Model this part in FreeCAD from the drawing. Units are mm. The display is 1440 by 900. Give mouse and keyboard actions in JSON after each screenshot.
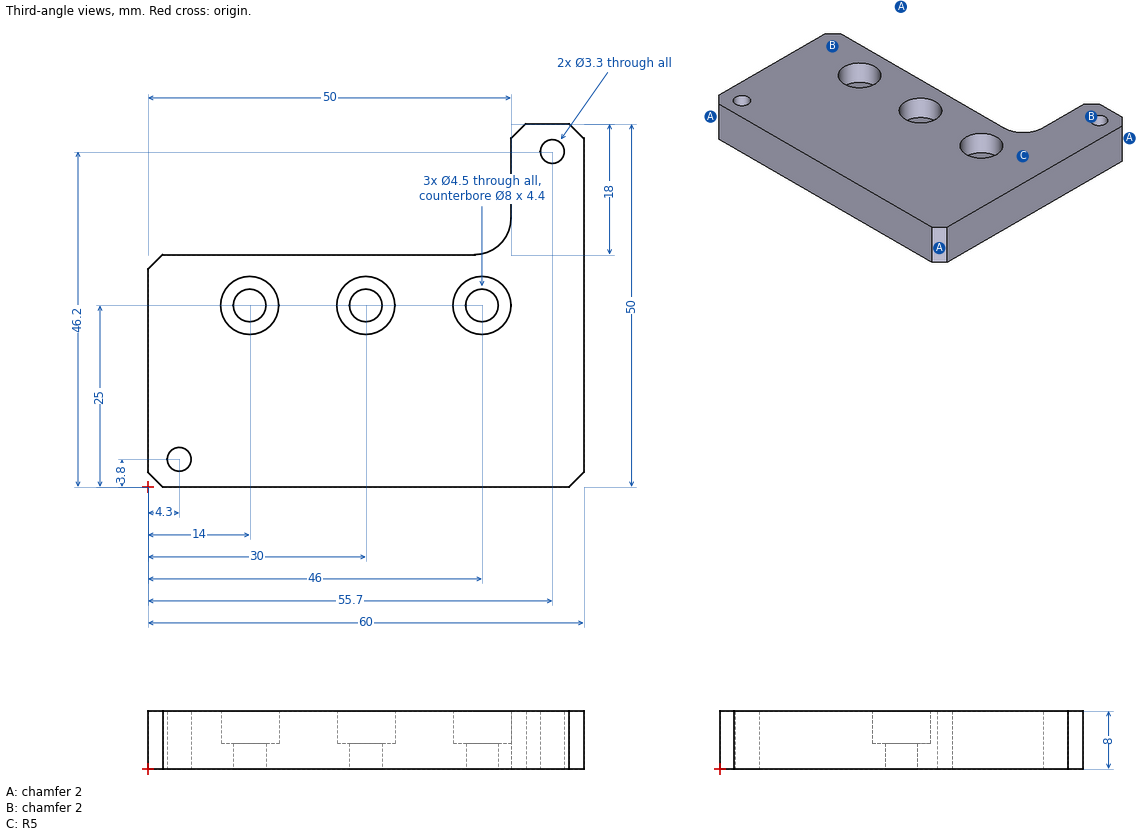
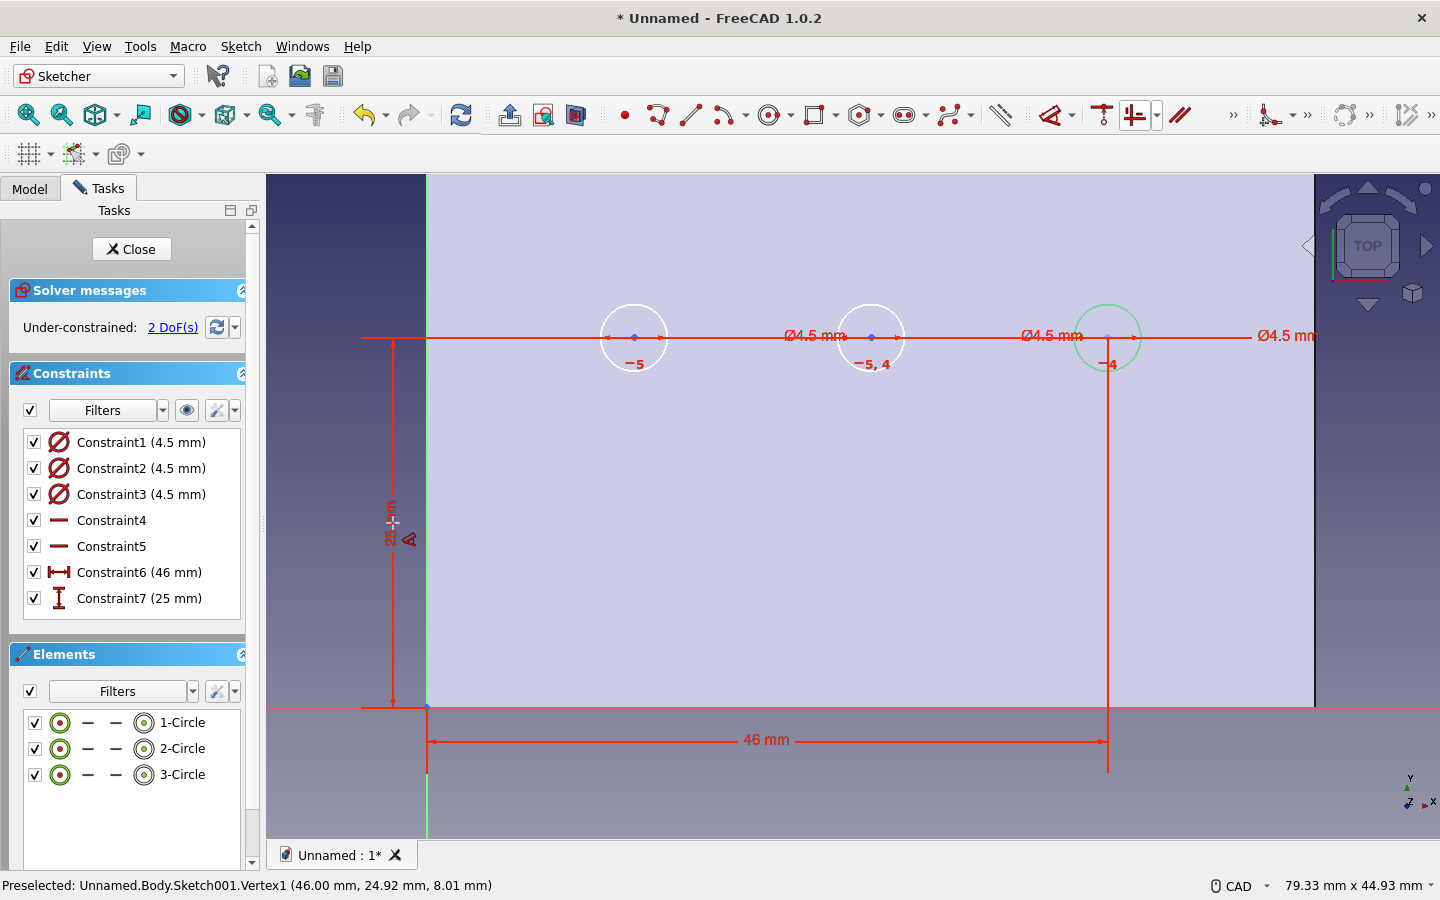
{"action": "left_click", "coordinate": [871, 338]}
{"action": "left_click", "coordinate": [649, 742]}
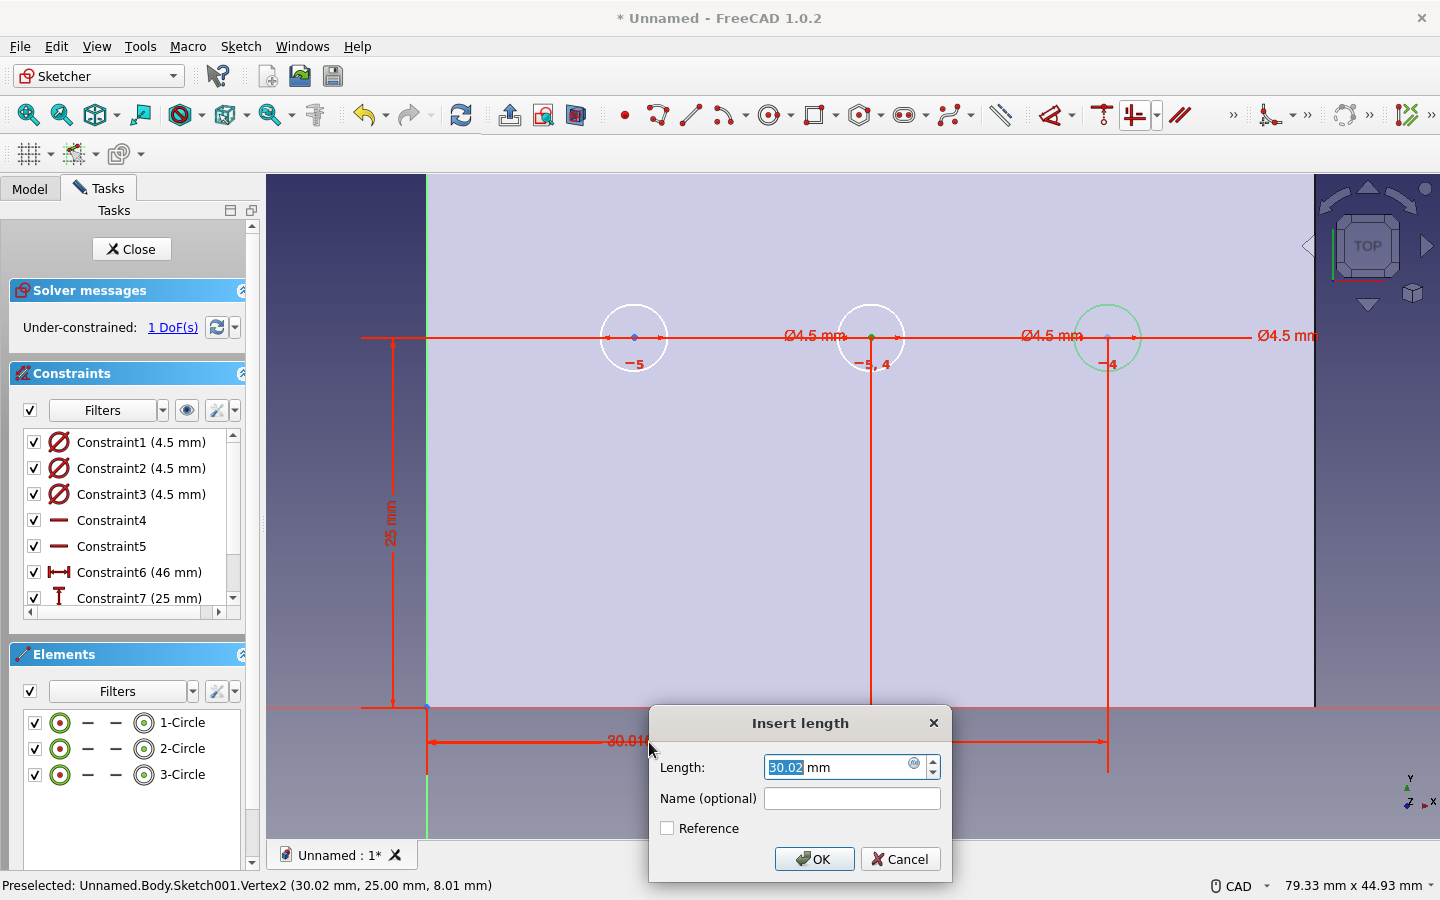
{"action": "type", "text": "30"}
{"action": "key", "text": "Return"}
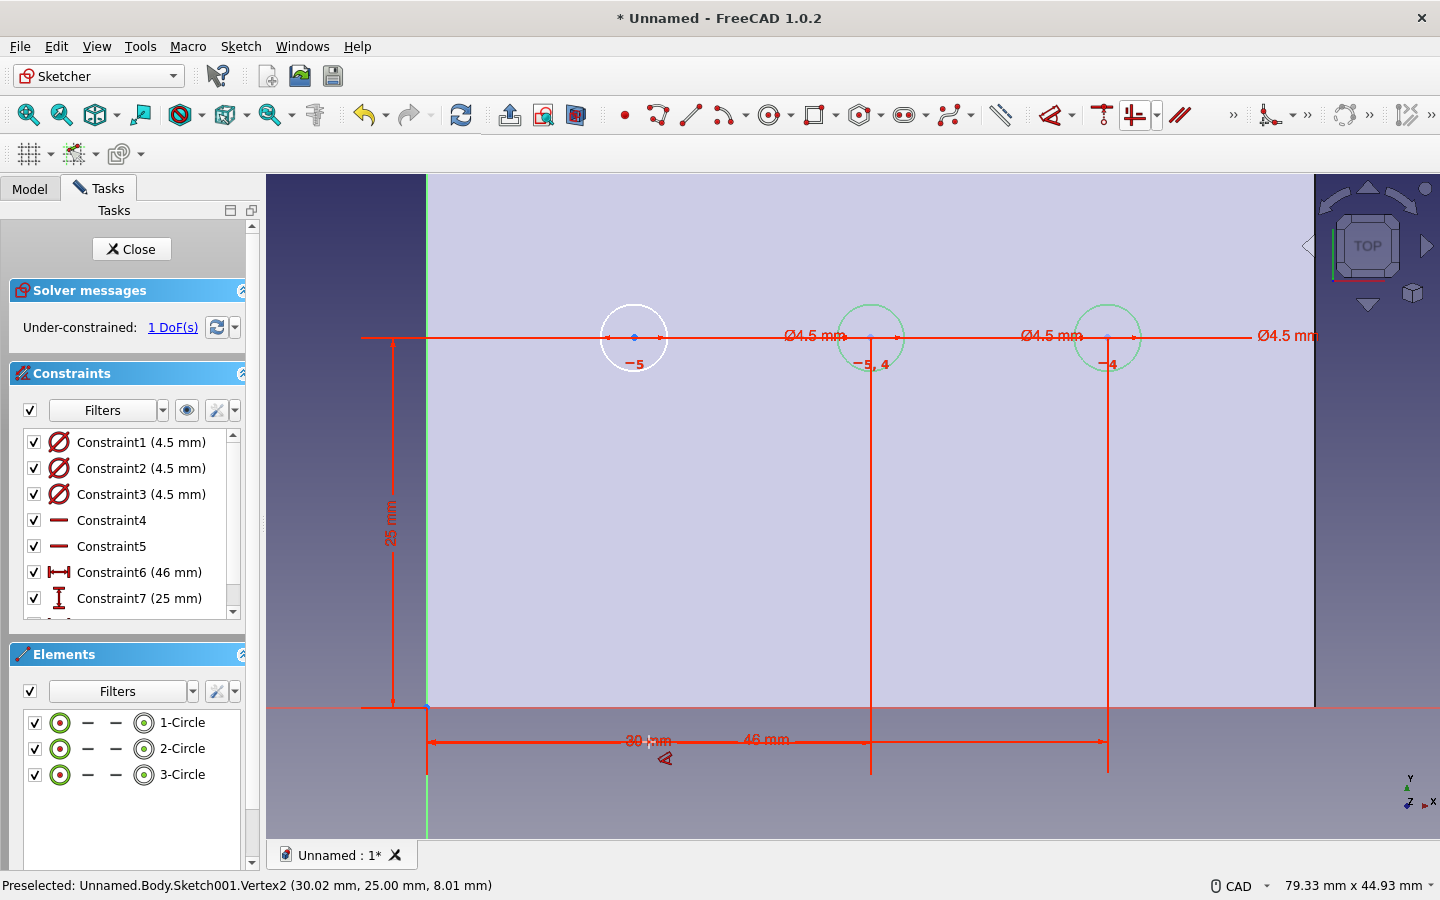
{"action": "left_click", "coordinate": [634, 338]}
{"action": "left_click", "coordinate": [530, 742]}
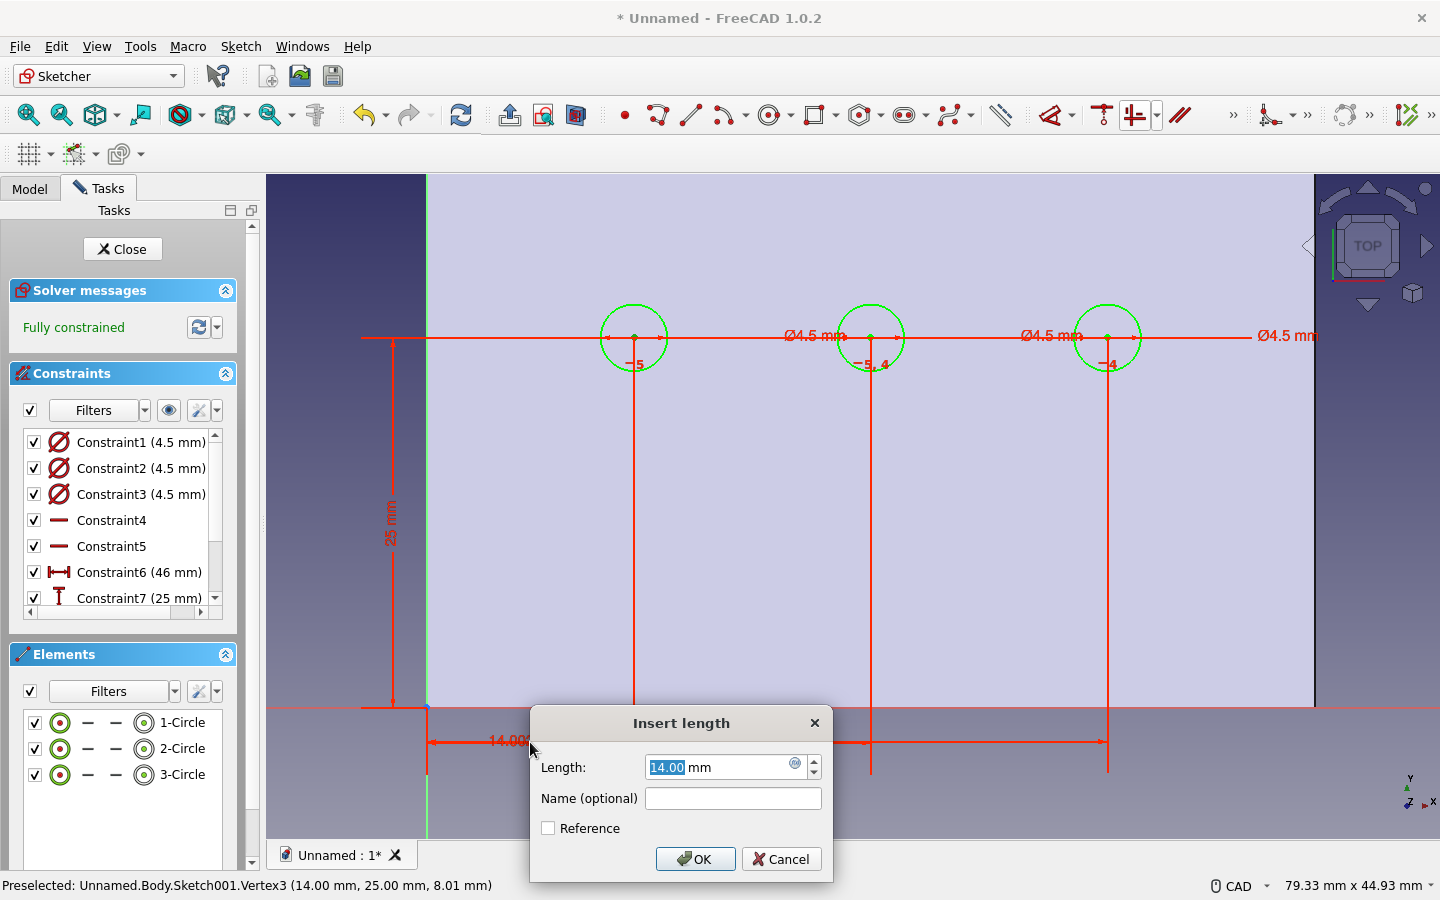
{"action": "type", "text": "14"}
{"action": "key", "text": "Return"}
{"action": "key", "text": "Escape"}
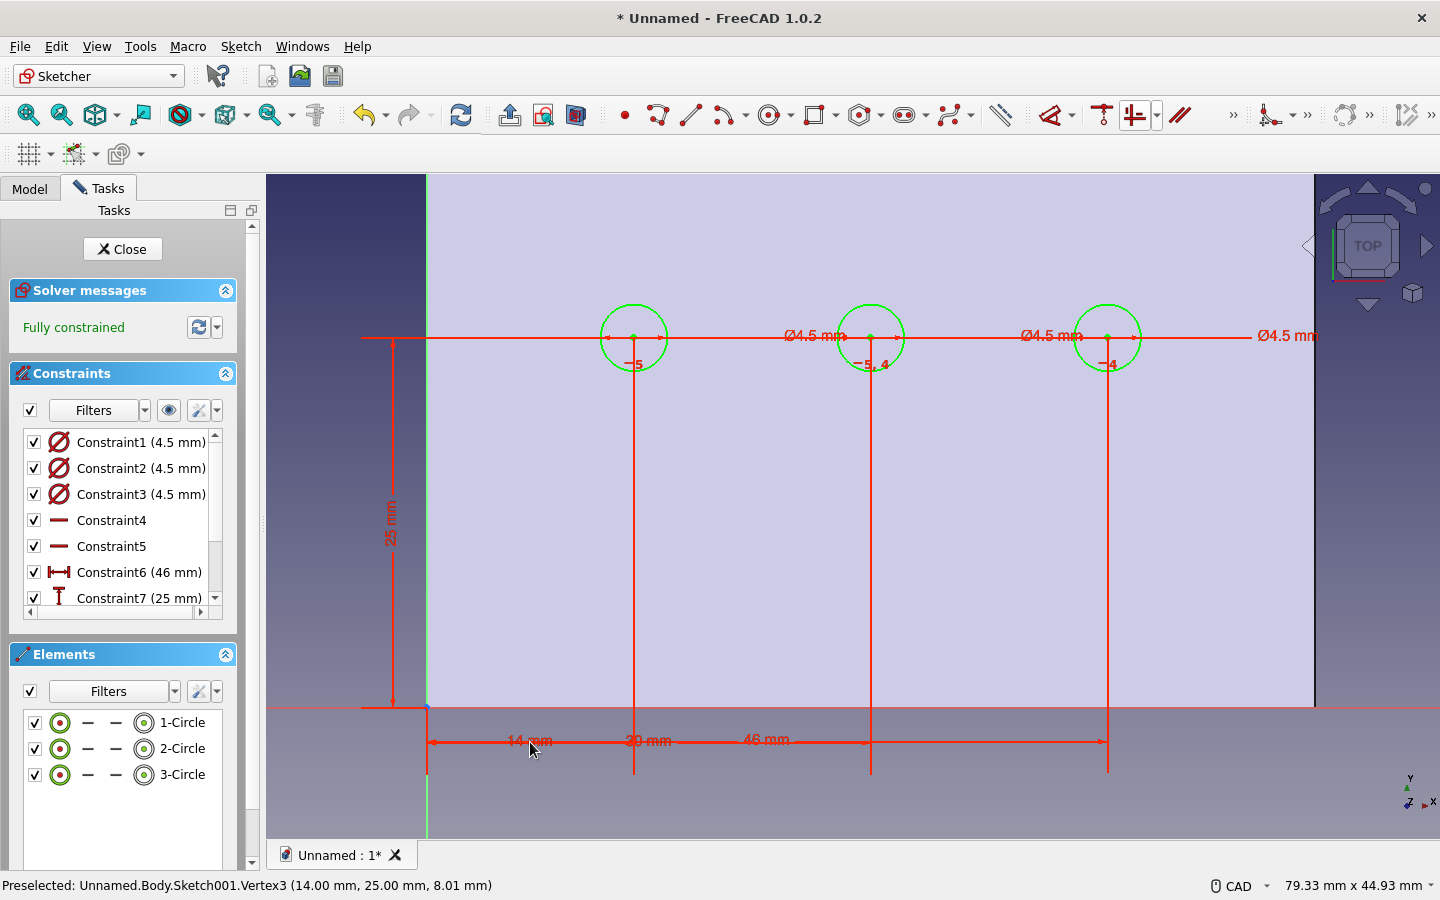
{"action": "left_click", "coordinate": [123, 249]}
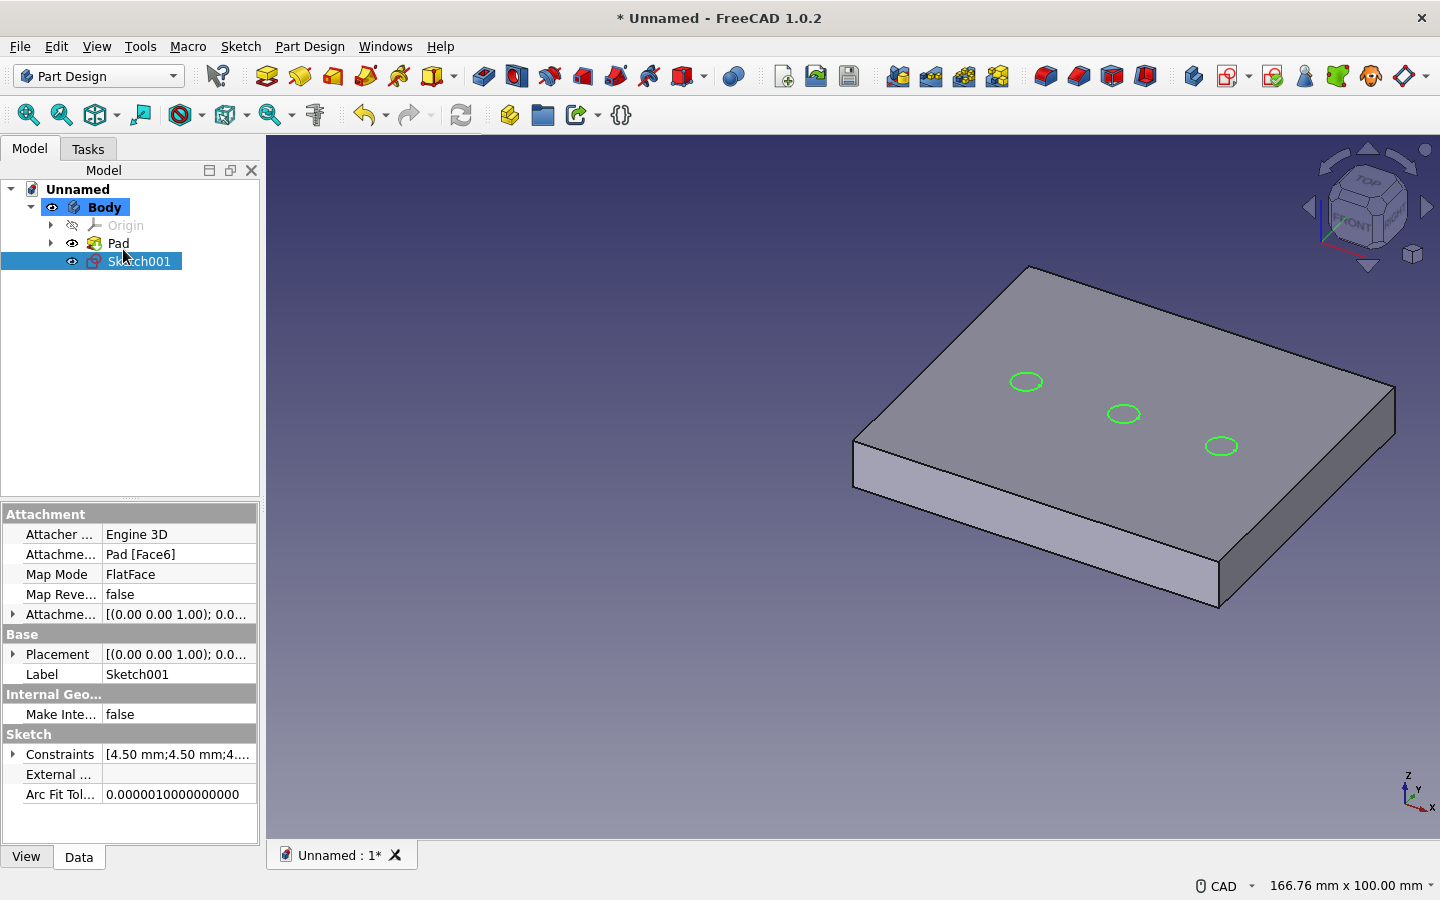
{"action": "left_click", "coordinate": [517, 76]}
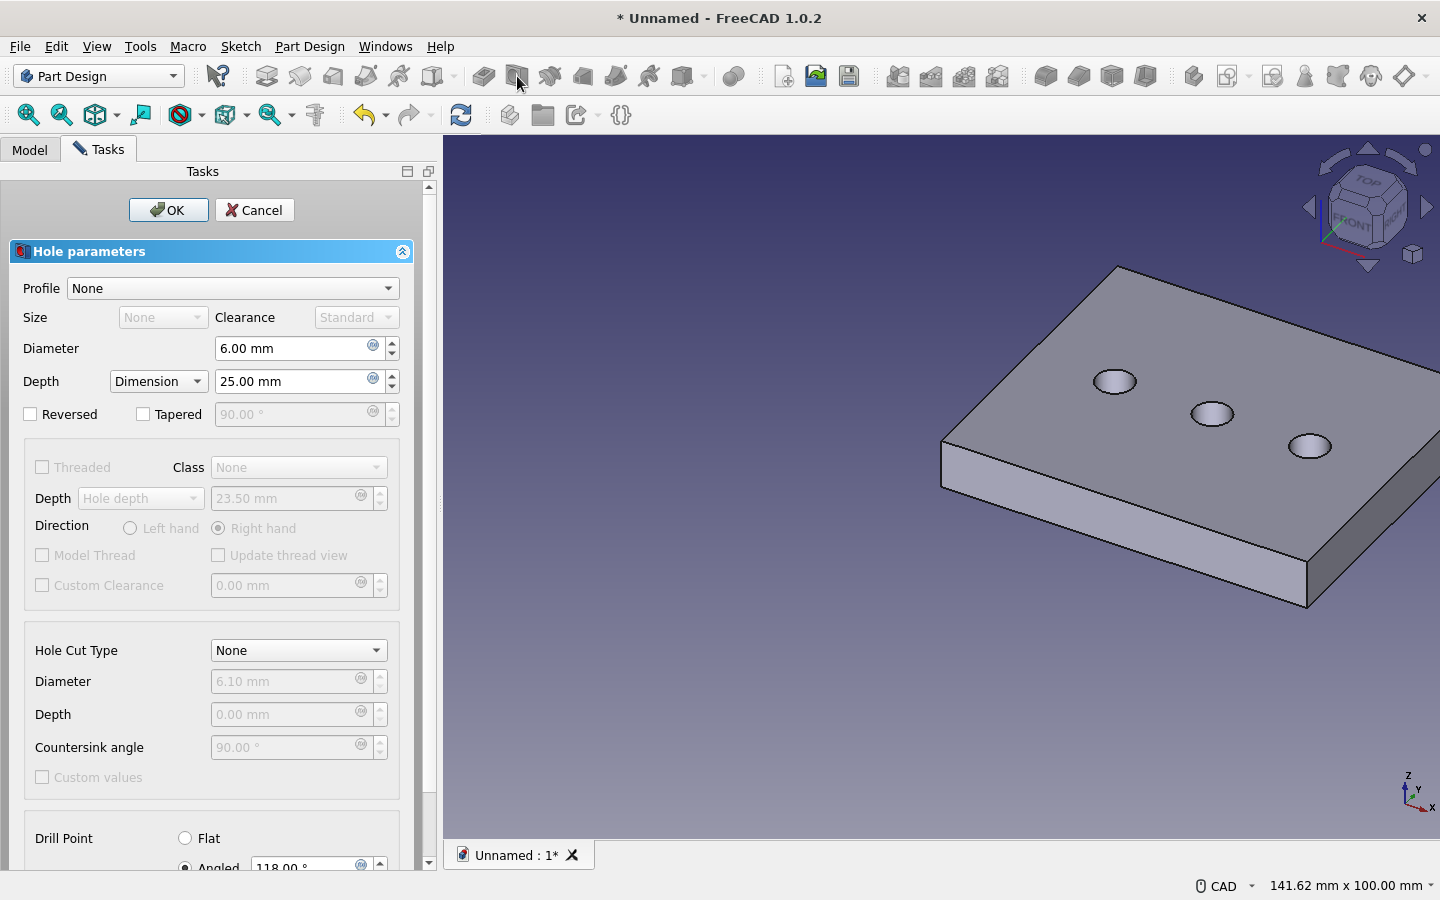
{"action": "triple_click", "coordinate": [300, 348]}